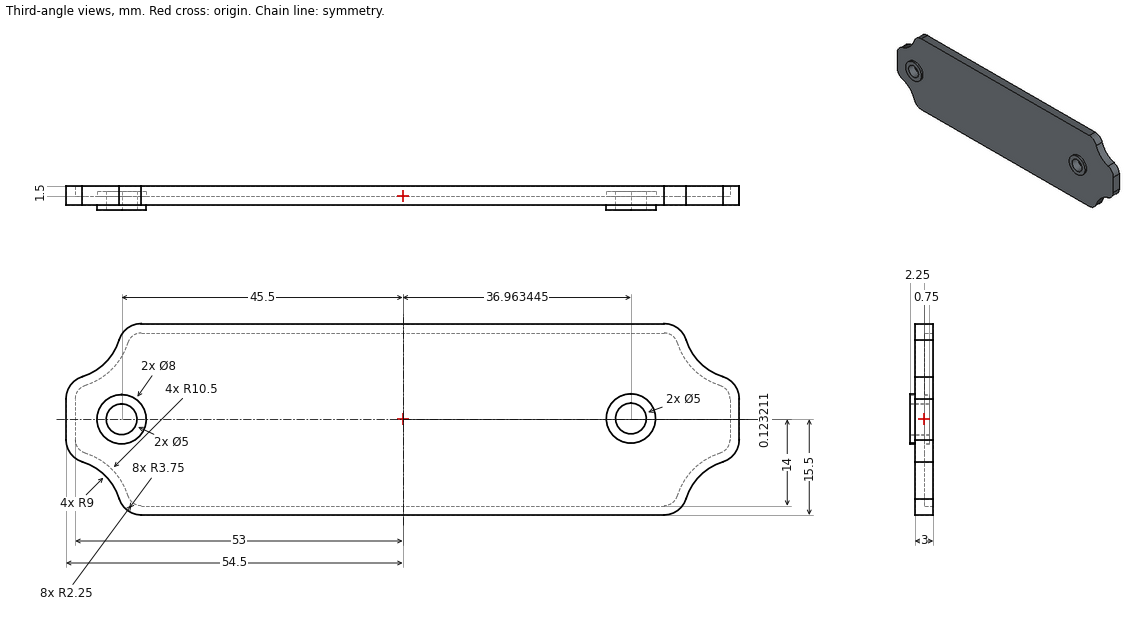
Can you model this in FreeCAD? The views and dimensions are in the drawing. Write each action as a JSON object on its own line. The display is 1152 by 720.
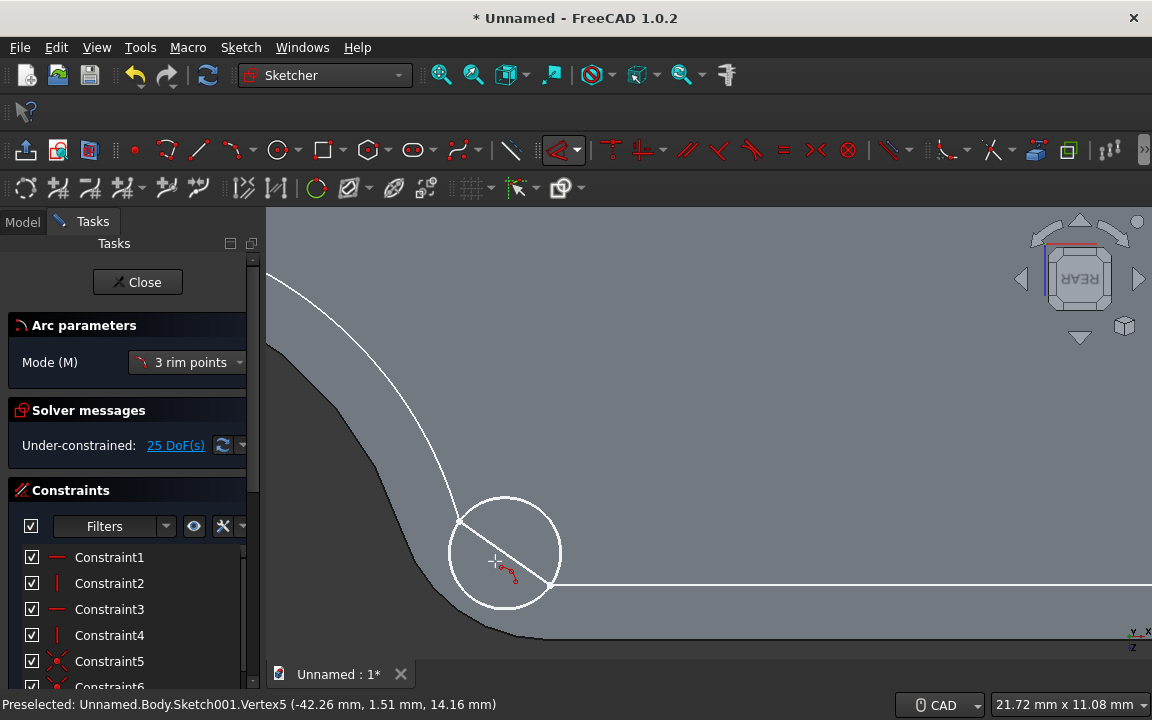
{"action": "left_click", "coordinate": [494, 561]}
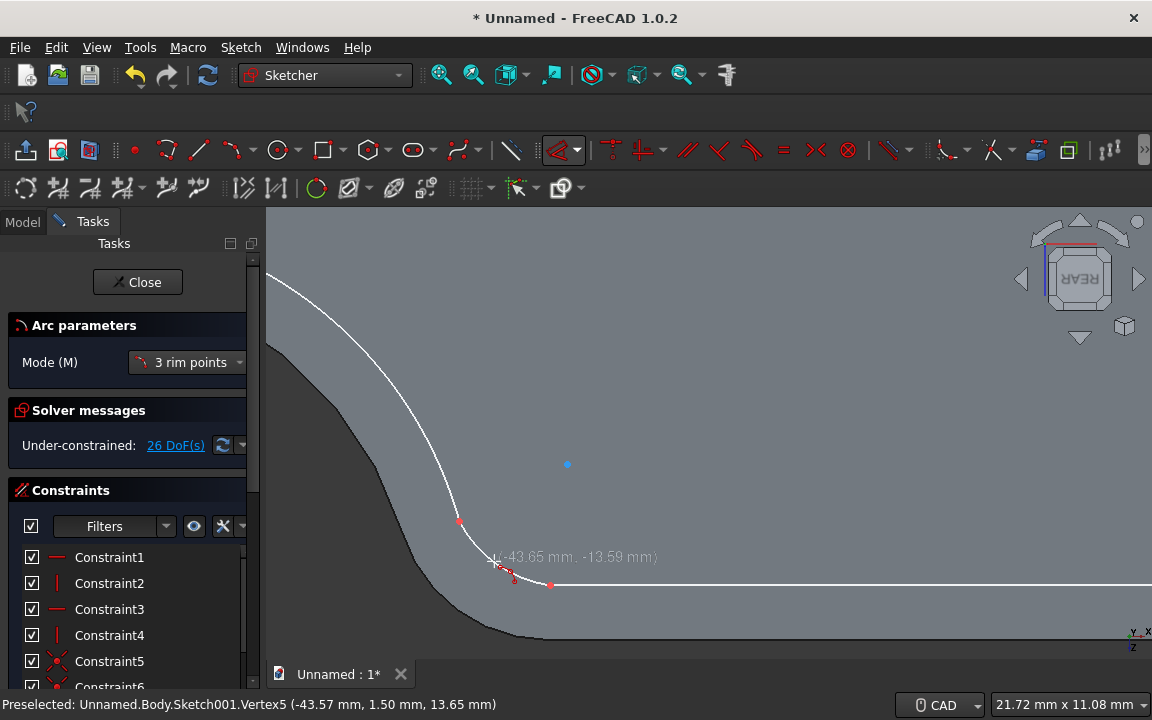
{"action": "scroll", "coordinate": [437, 486], "scroll_direction": "down", "scroll_amount": 11}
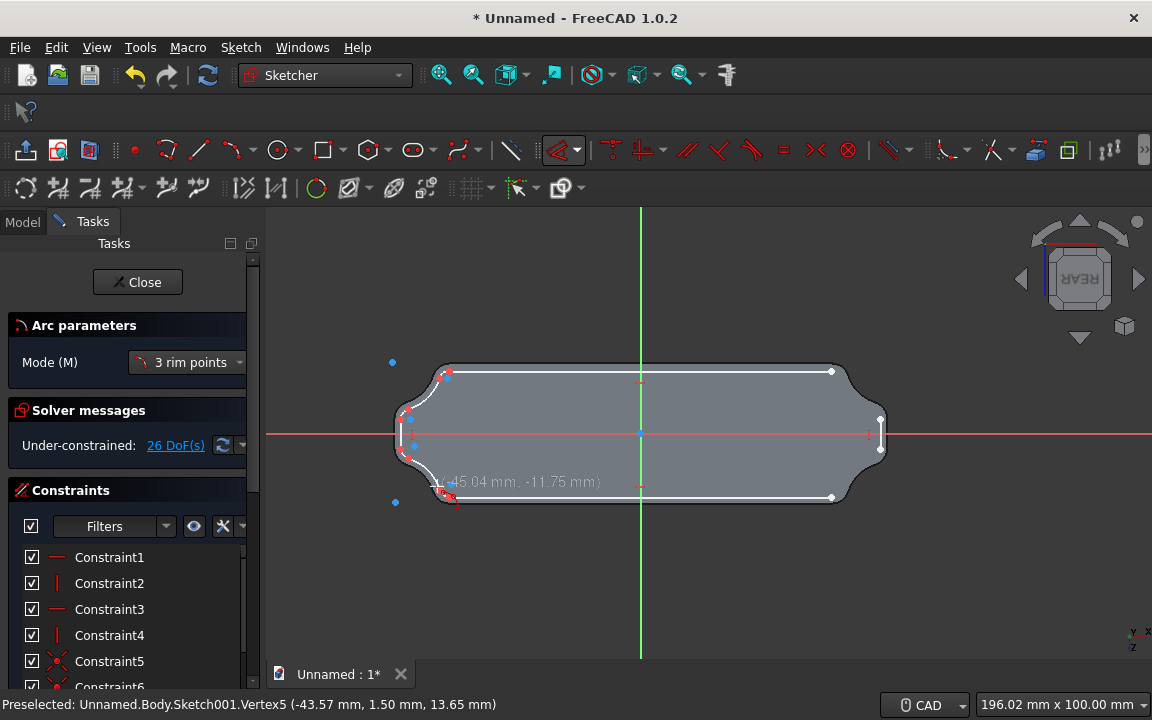
{"action": "left_click", "coordinate": [832, 498]}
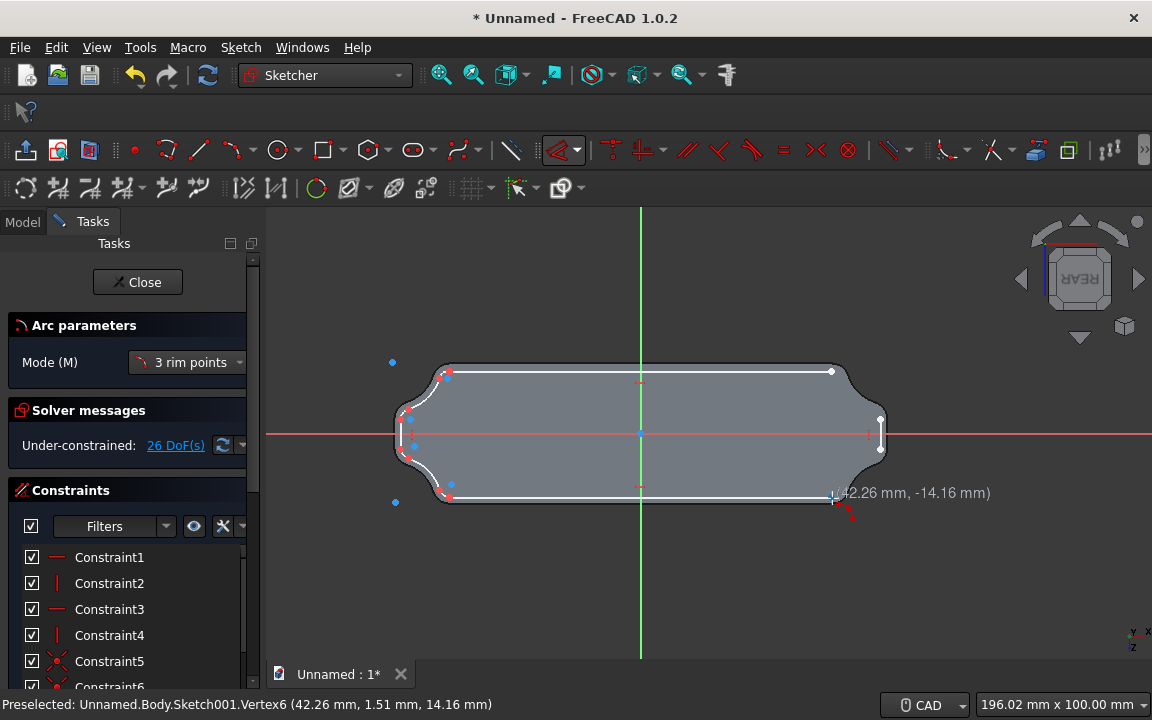
{"action": "scroll", "coordinate": [842, 490], "scroll_direction": "up", "scroll_amount": 2}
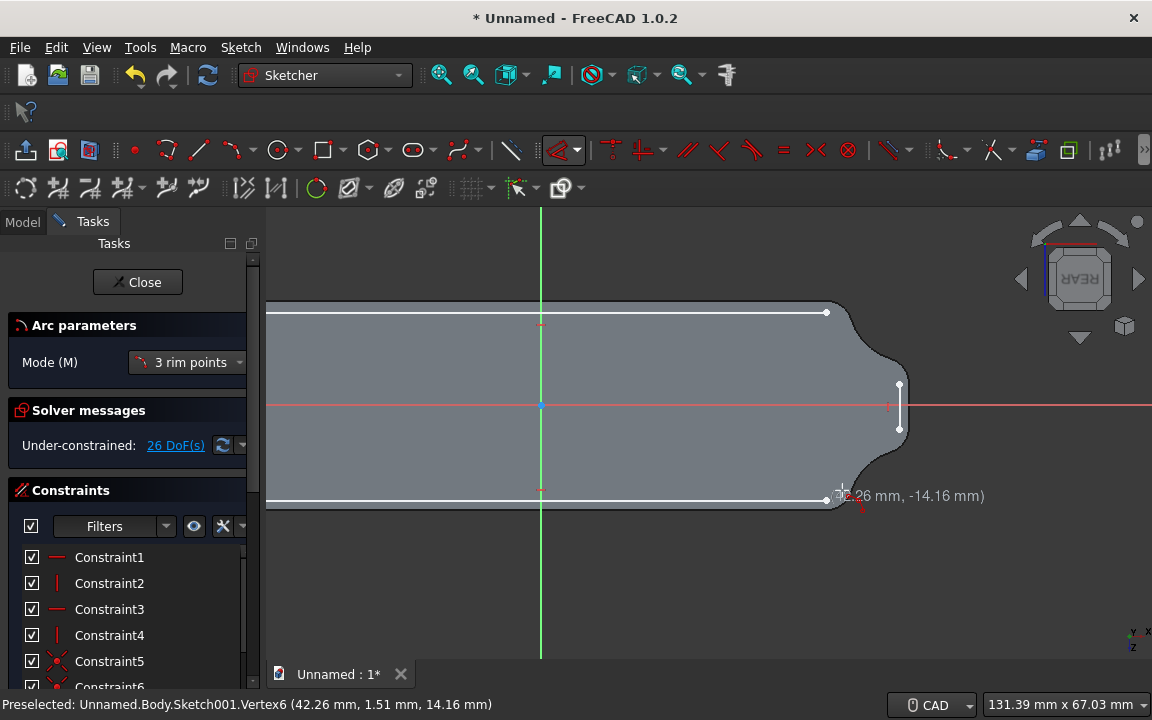
{"action": "left_click", "coordinate": [841, 489]}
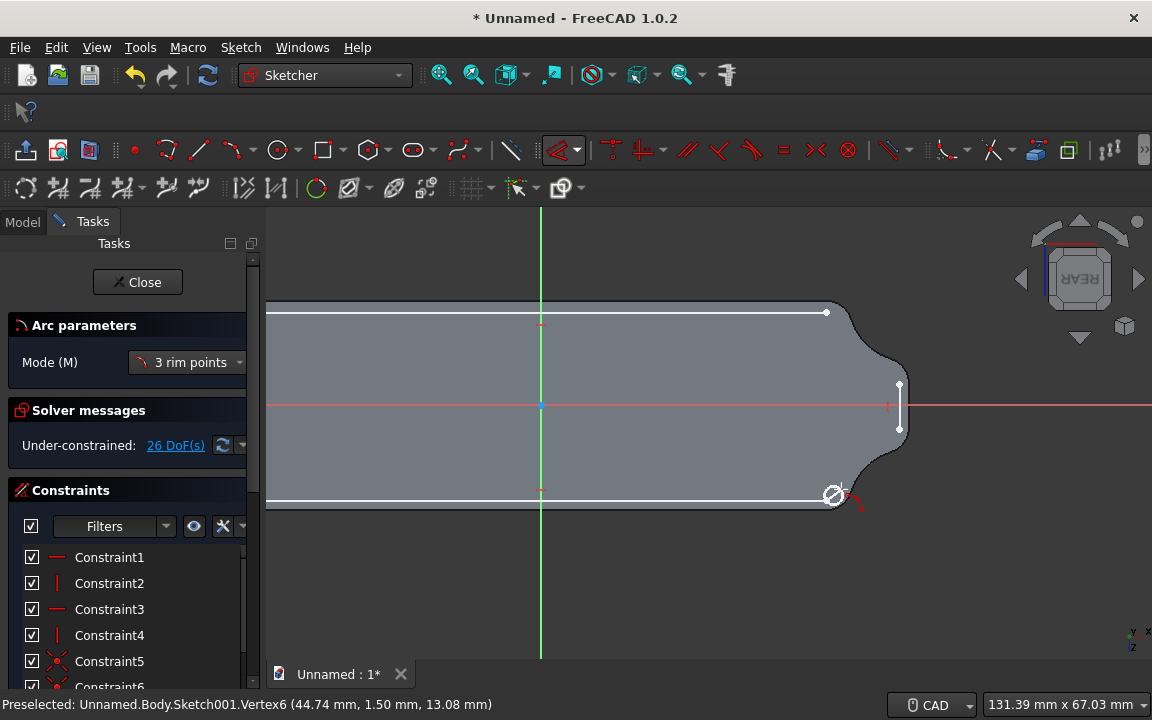
{"action": "scroll", "coordinate": [836, 497], "scroll_direction": "up", "scroll_amount": 9}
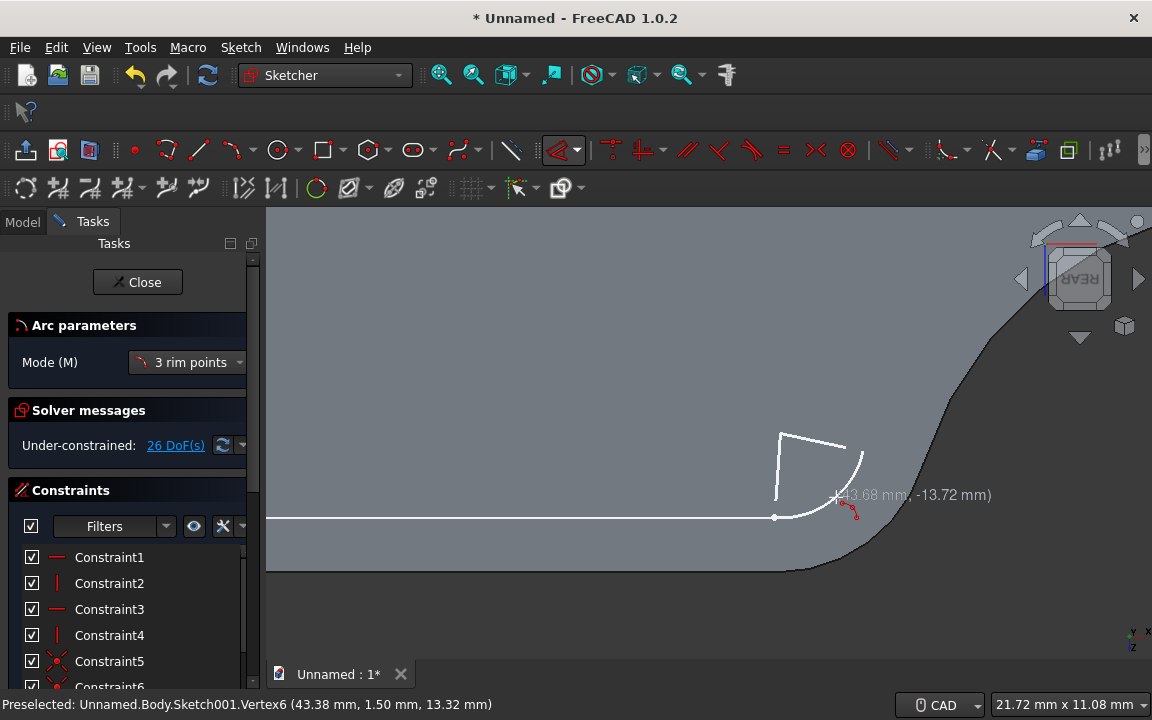
{"action": "left_click", "coordinate": [832, 493]}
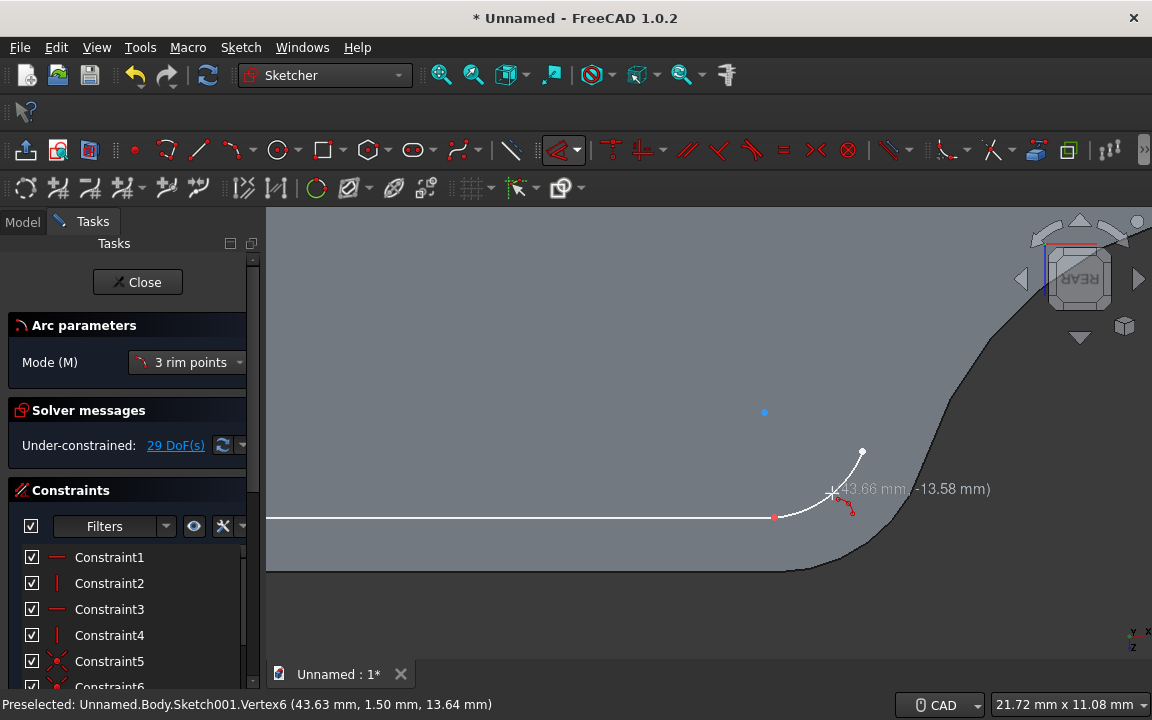
{"action": "scroll", "coordinate": [839, 494], "scroll_direction": "down", "scroll_amount": 11}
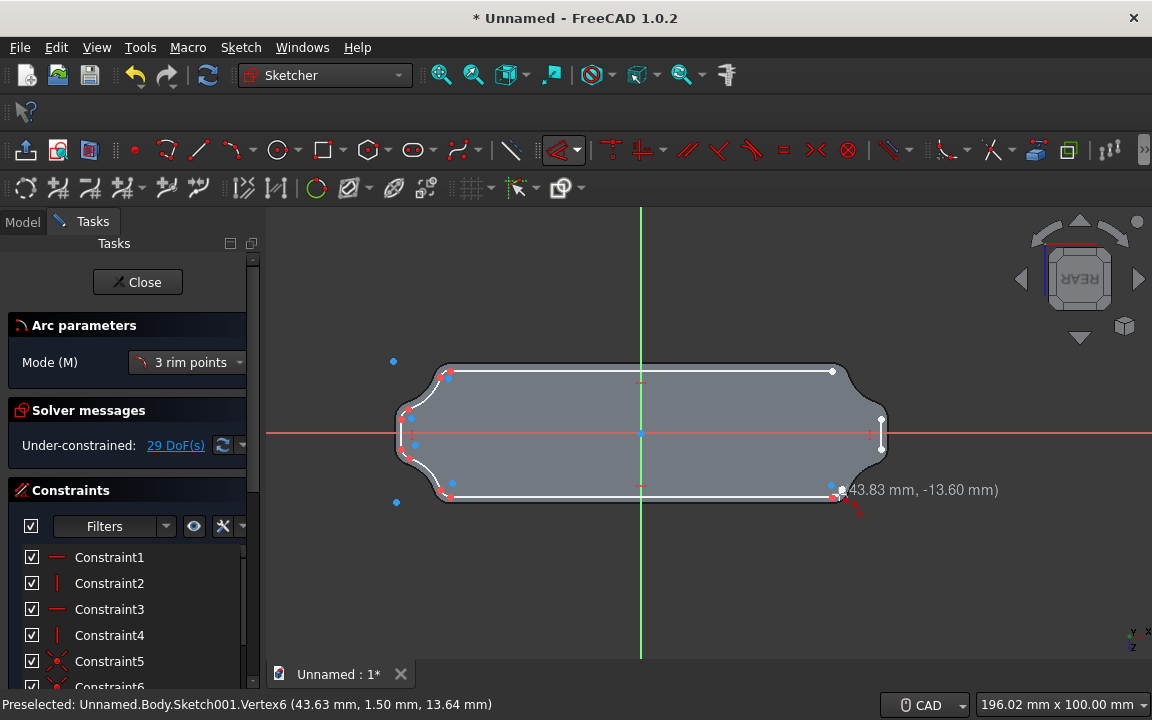
{"action": "scroll", "coordinate": [842, 489], "scroll_direction": "up", "scroll_amount": 3}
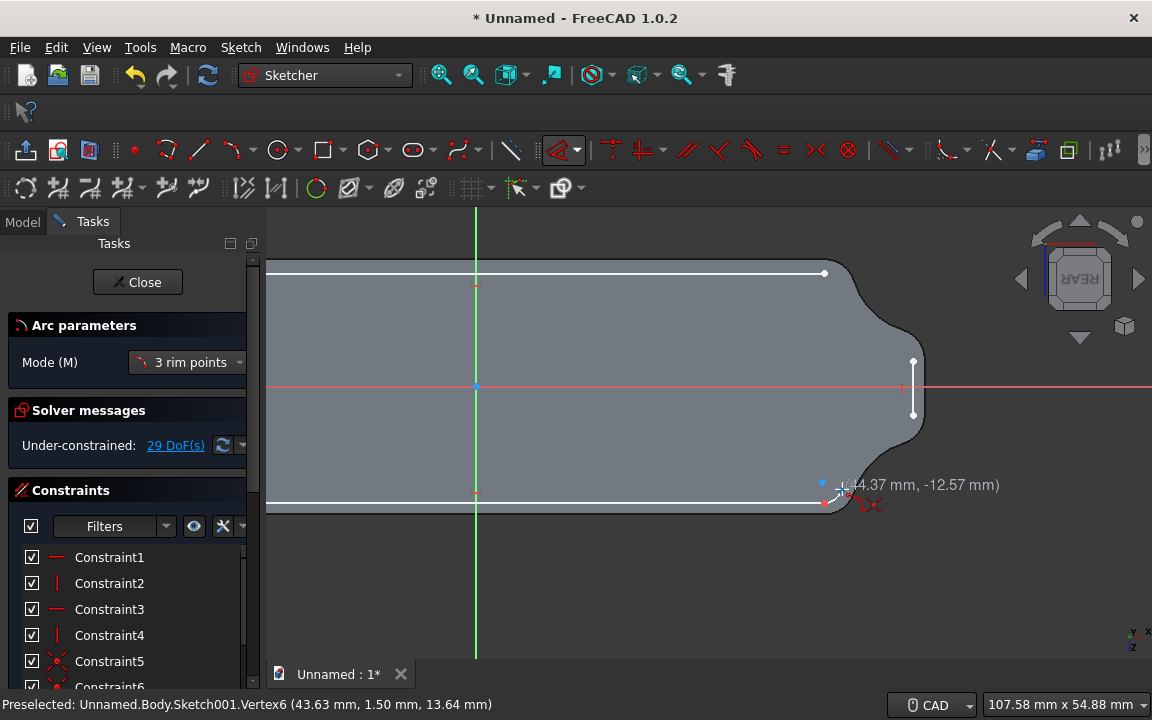
{"action": "left_click", "coordinate": [842, 490]}
{"action": "left_click", "coordinate": [899, 432]}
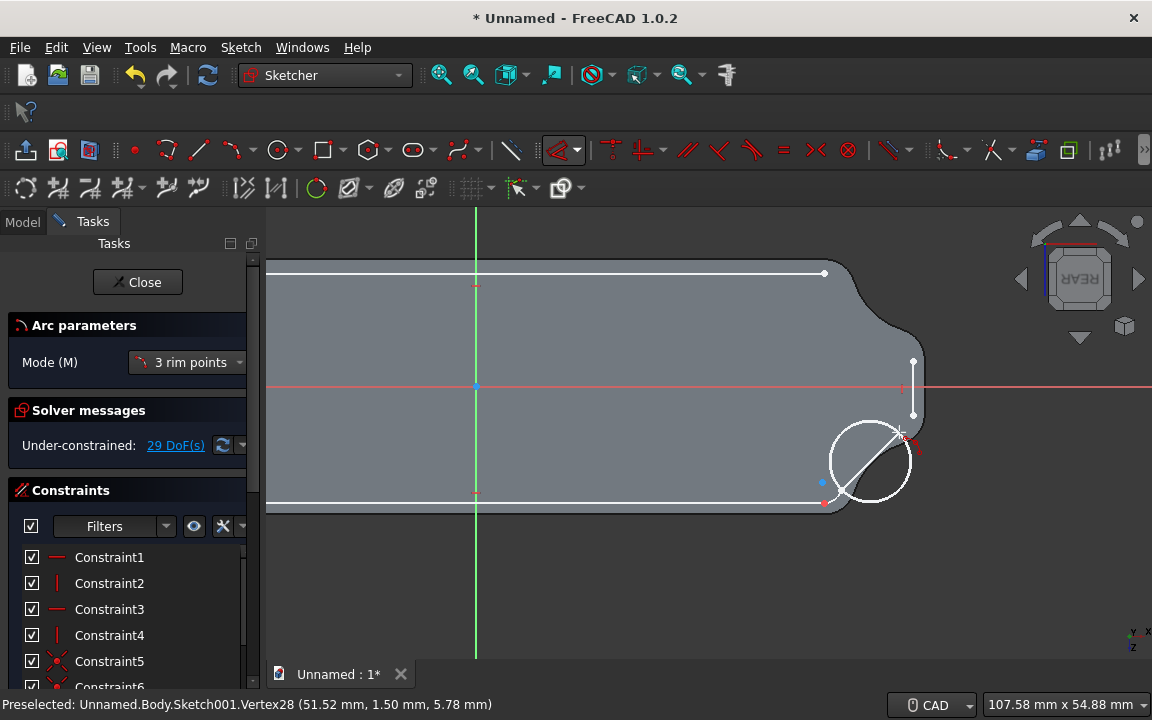
{"action": "scroll", "coordinate": [864, 453], "scroll_direction": "up", "scroll_amount": 3}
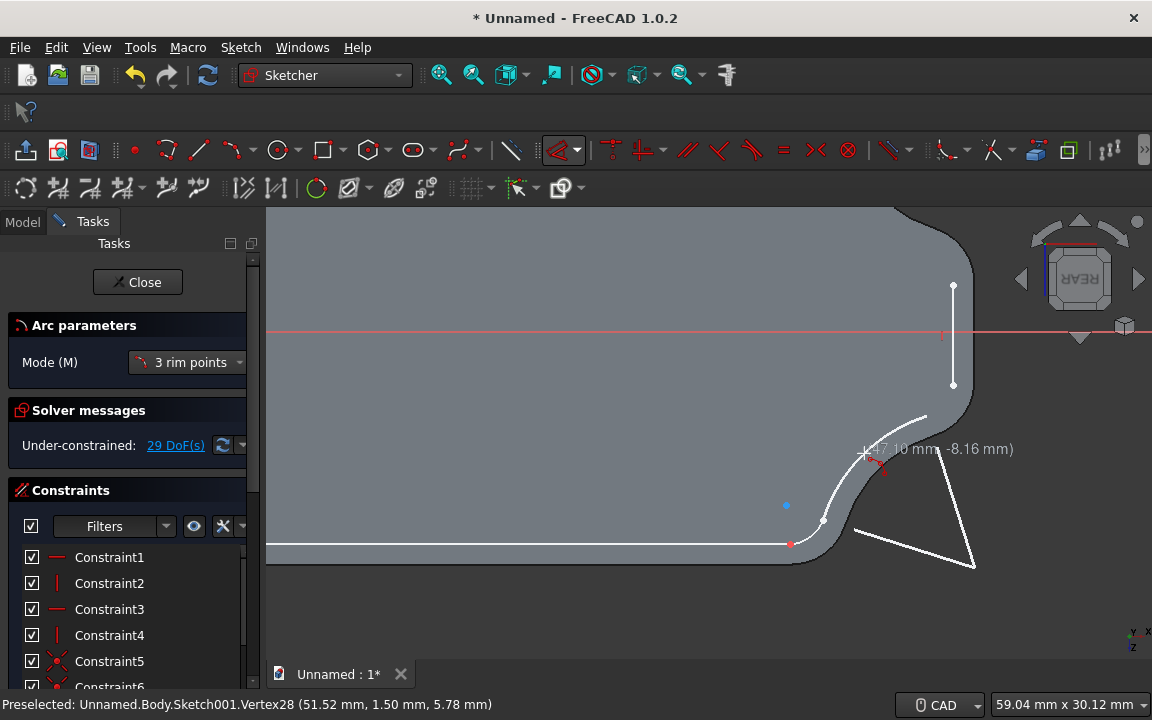
{"action": "left_click", "coordinate": [863, 453]}